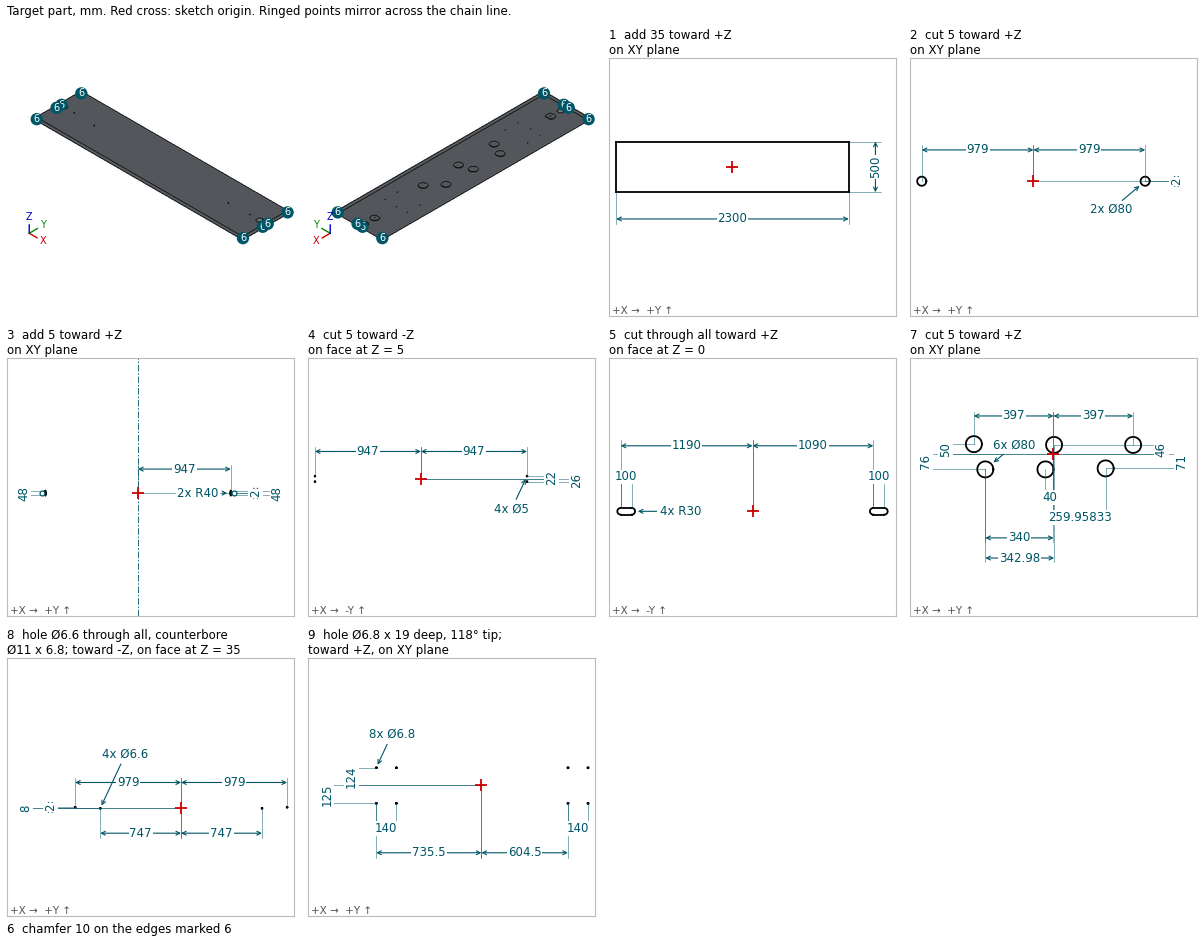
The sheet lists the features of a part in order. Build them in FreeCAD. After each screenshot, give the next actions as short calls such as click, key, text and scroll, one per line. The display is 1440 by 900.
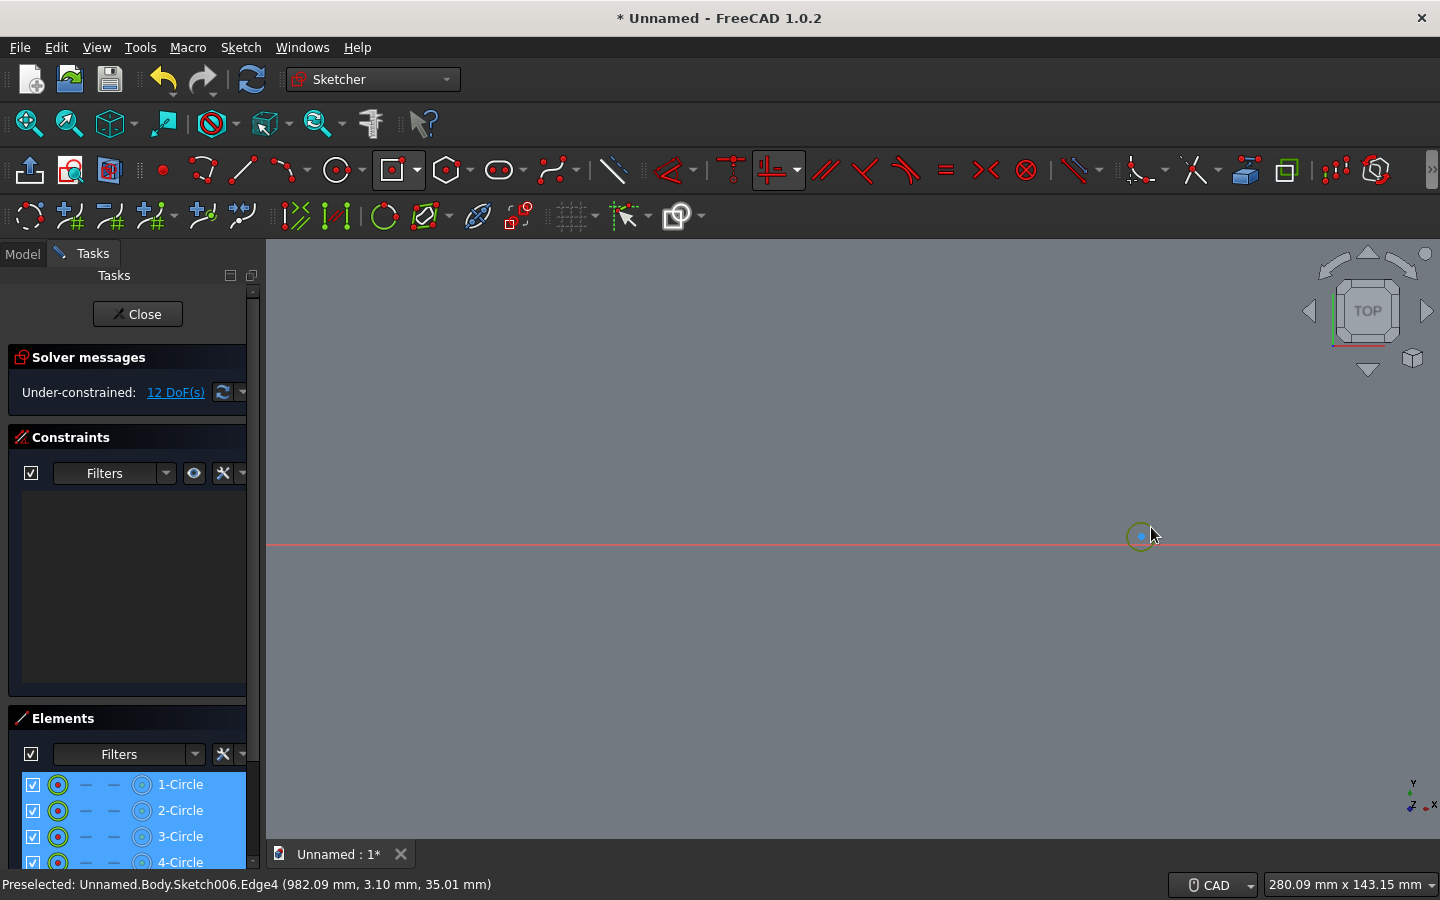
click(946, 170)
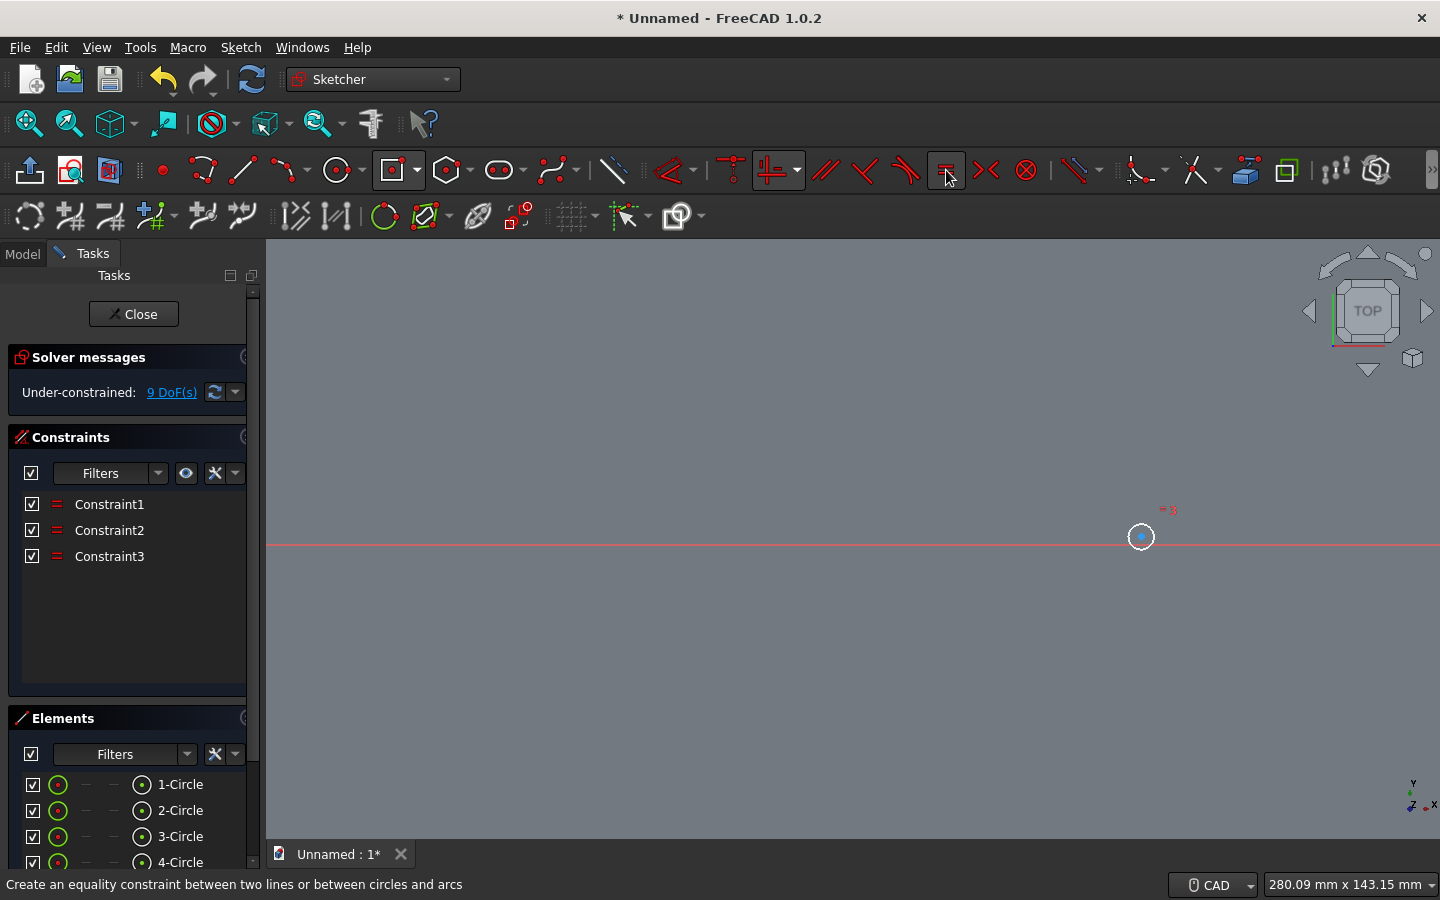
scroll(1158, 537, down, 12)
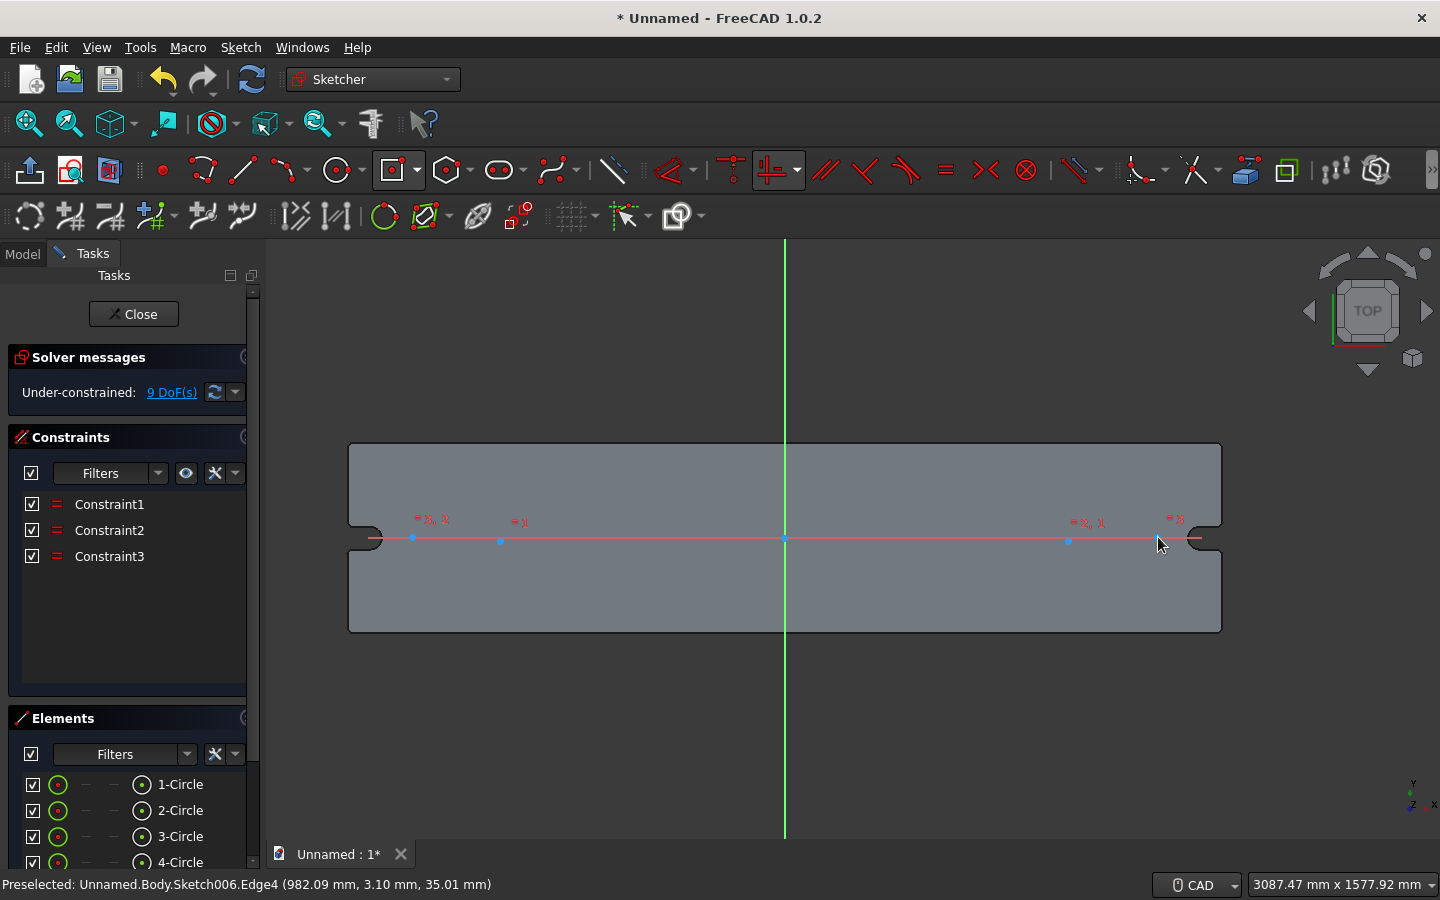
click(501, 541)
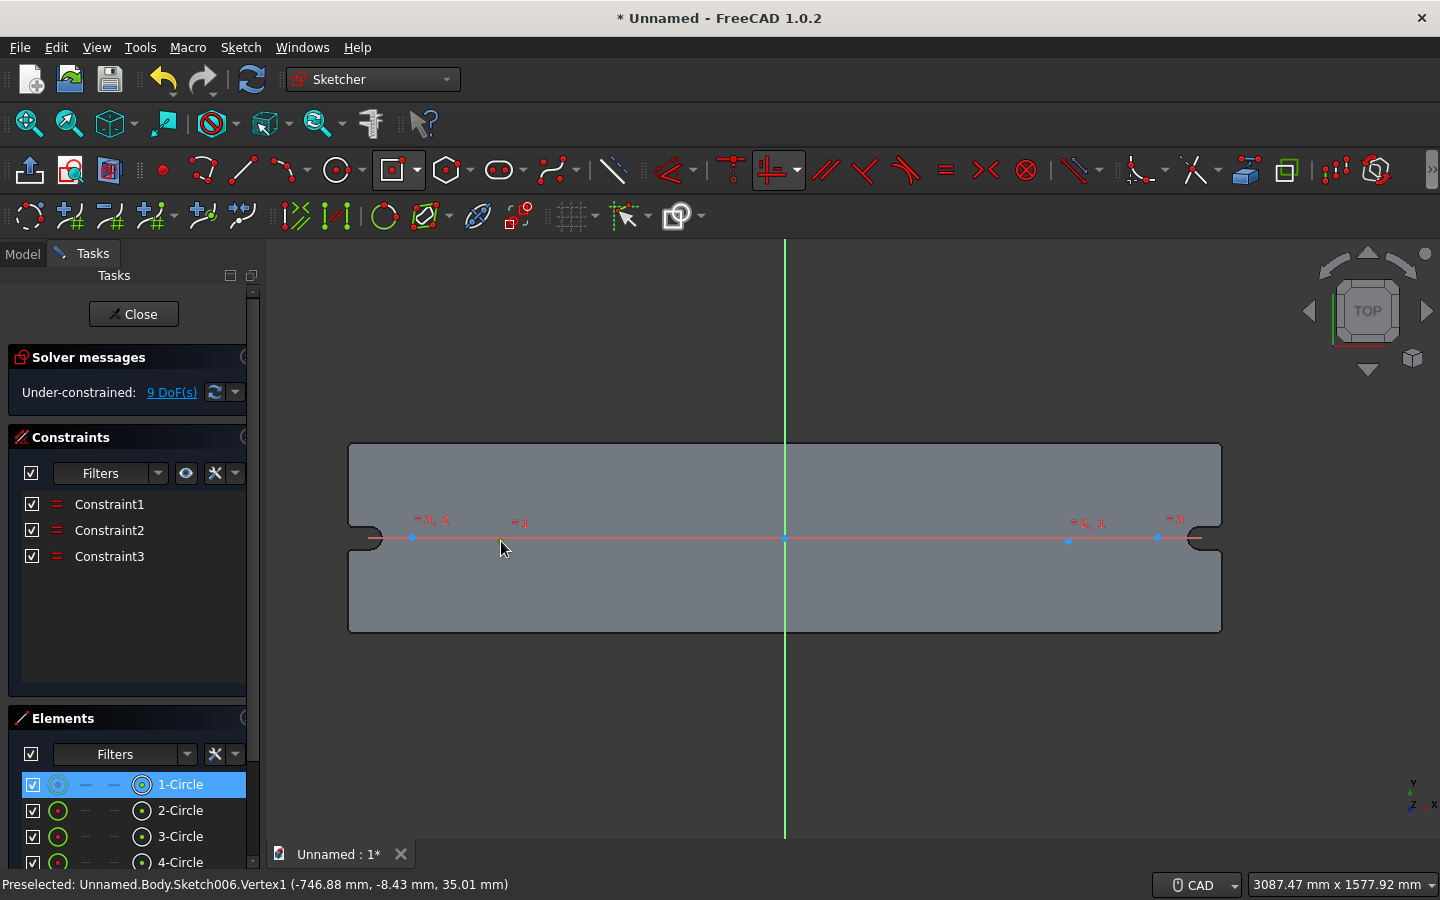
click(1069, 541)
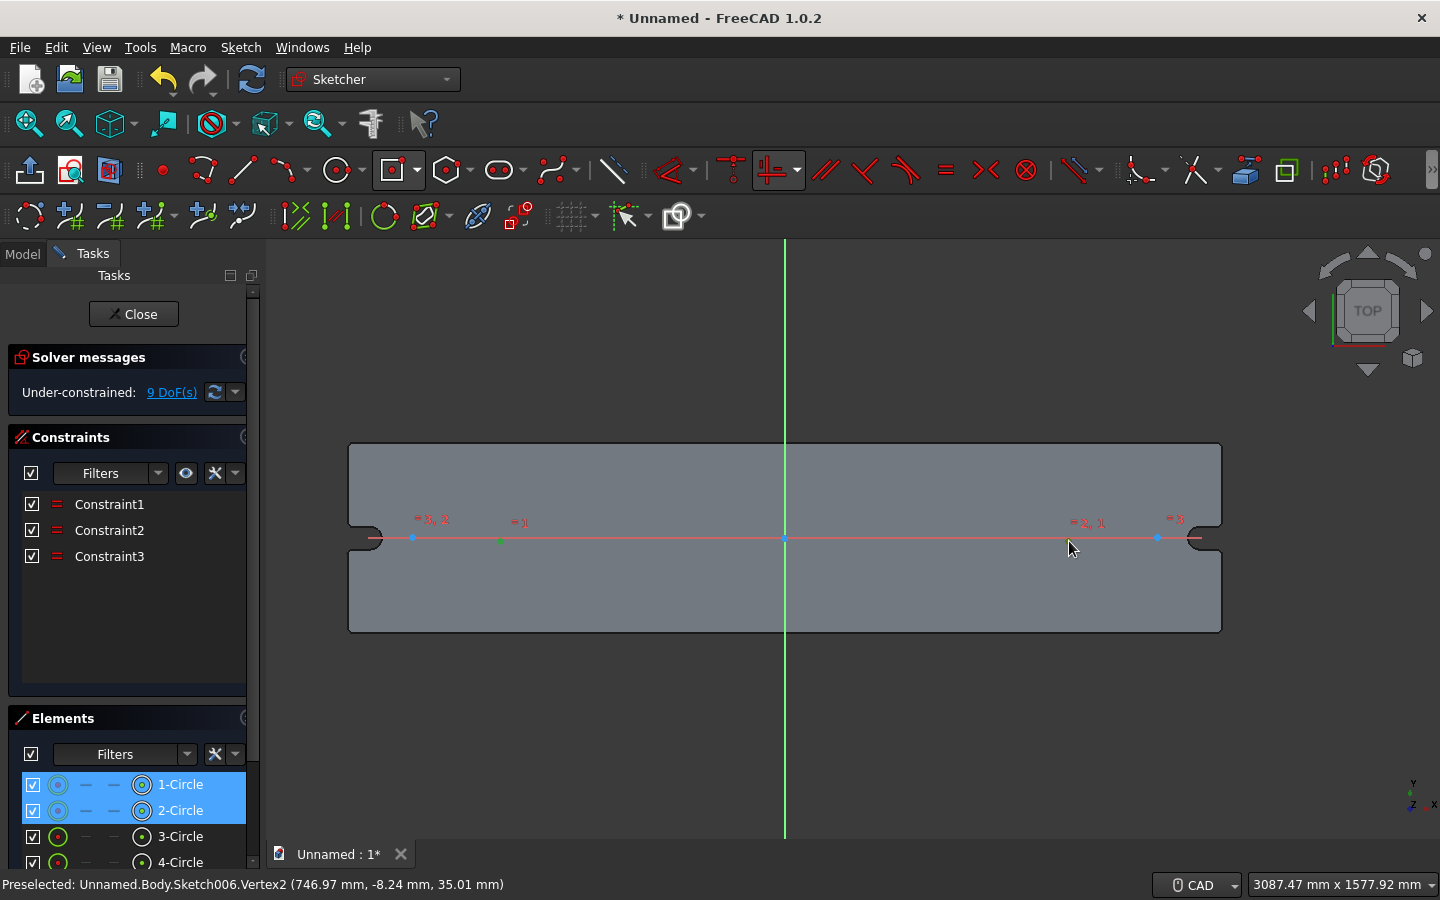
key(h)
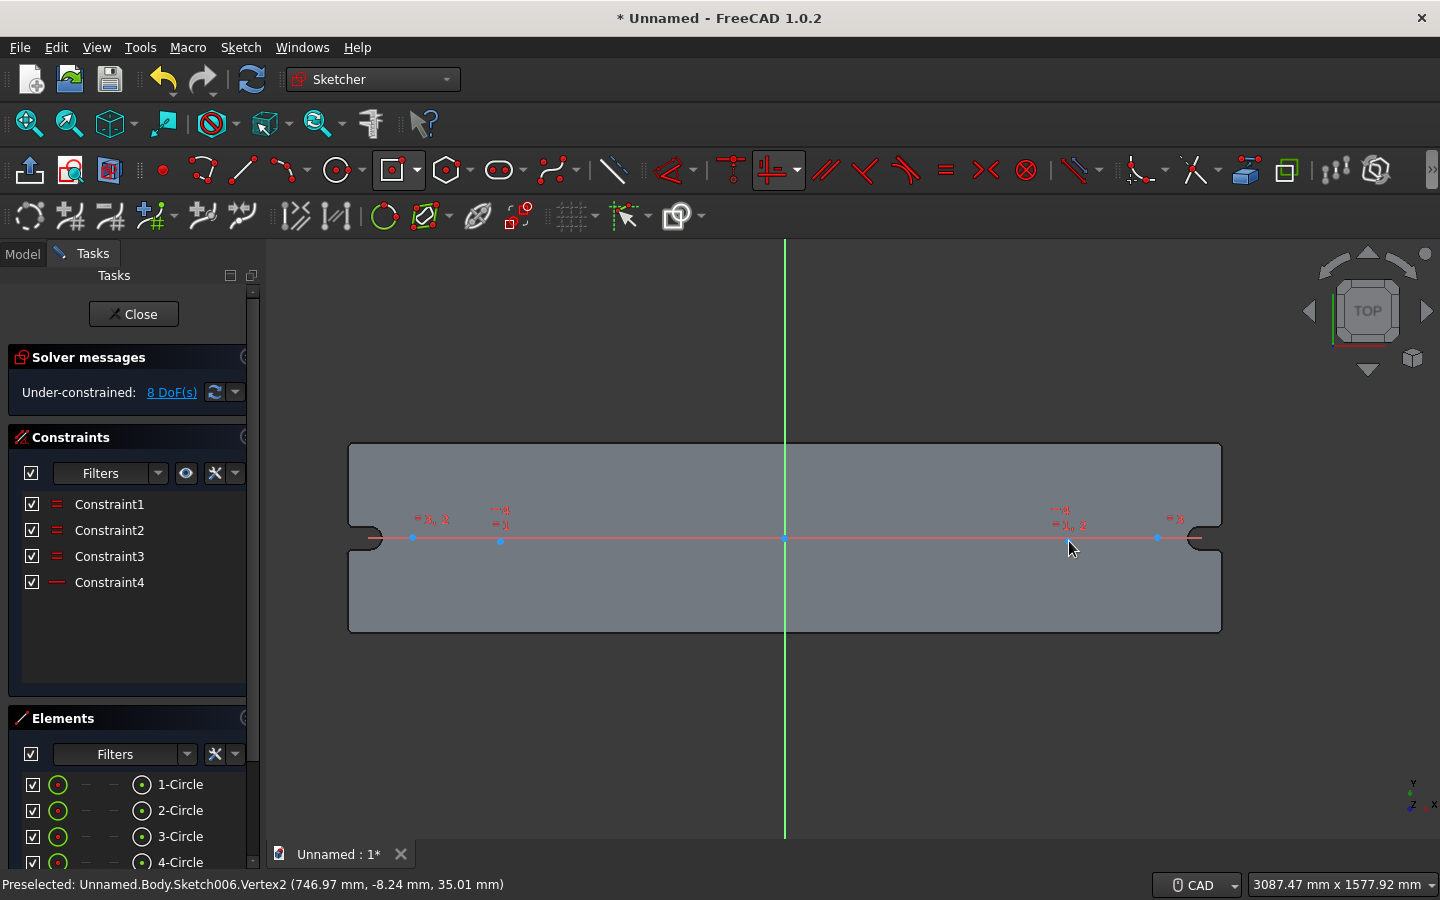
click(413, 537)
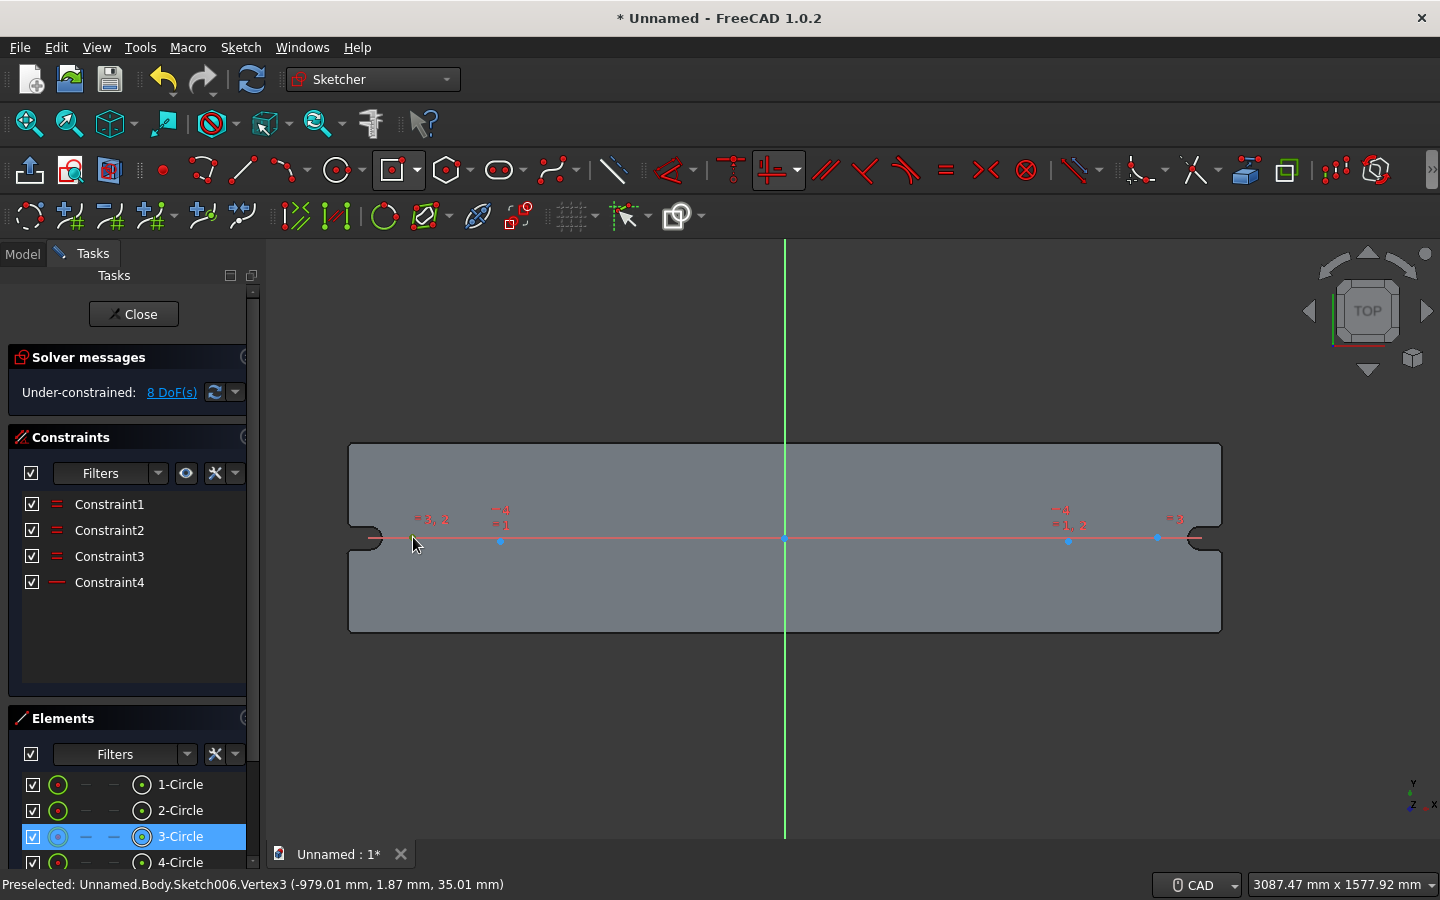
click(1157, 537)